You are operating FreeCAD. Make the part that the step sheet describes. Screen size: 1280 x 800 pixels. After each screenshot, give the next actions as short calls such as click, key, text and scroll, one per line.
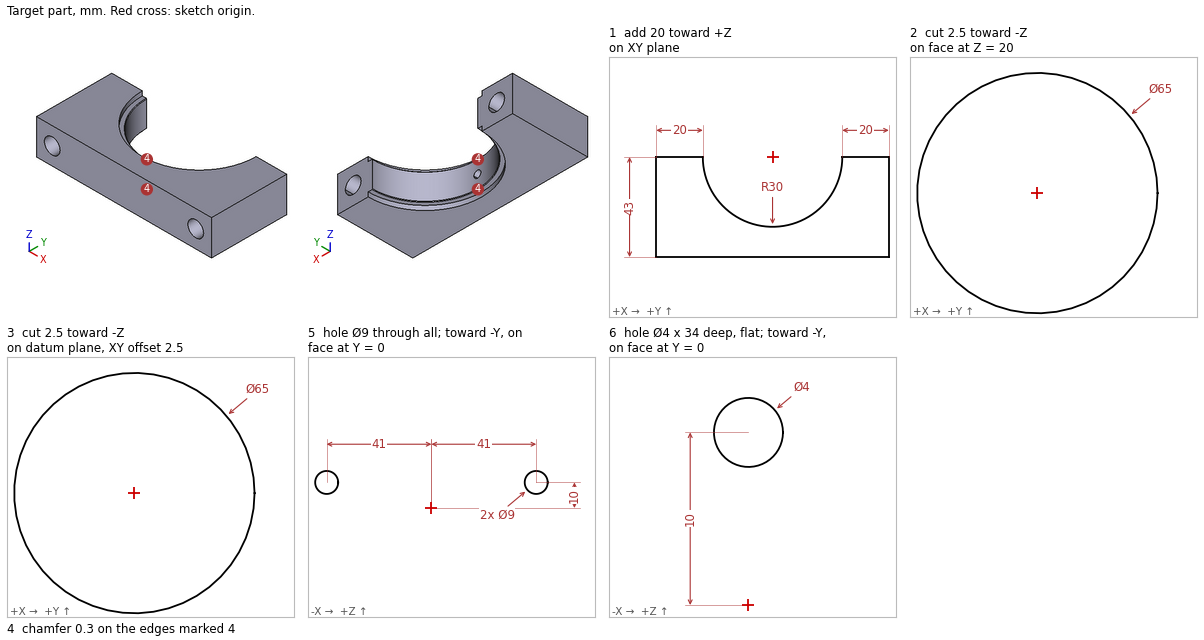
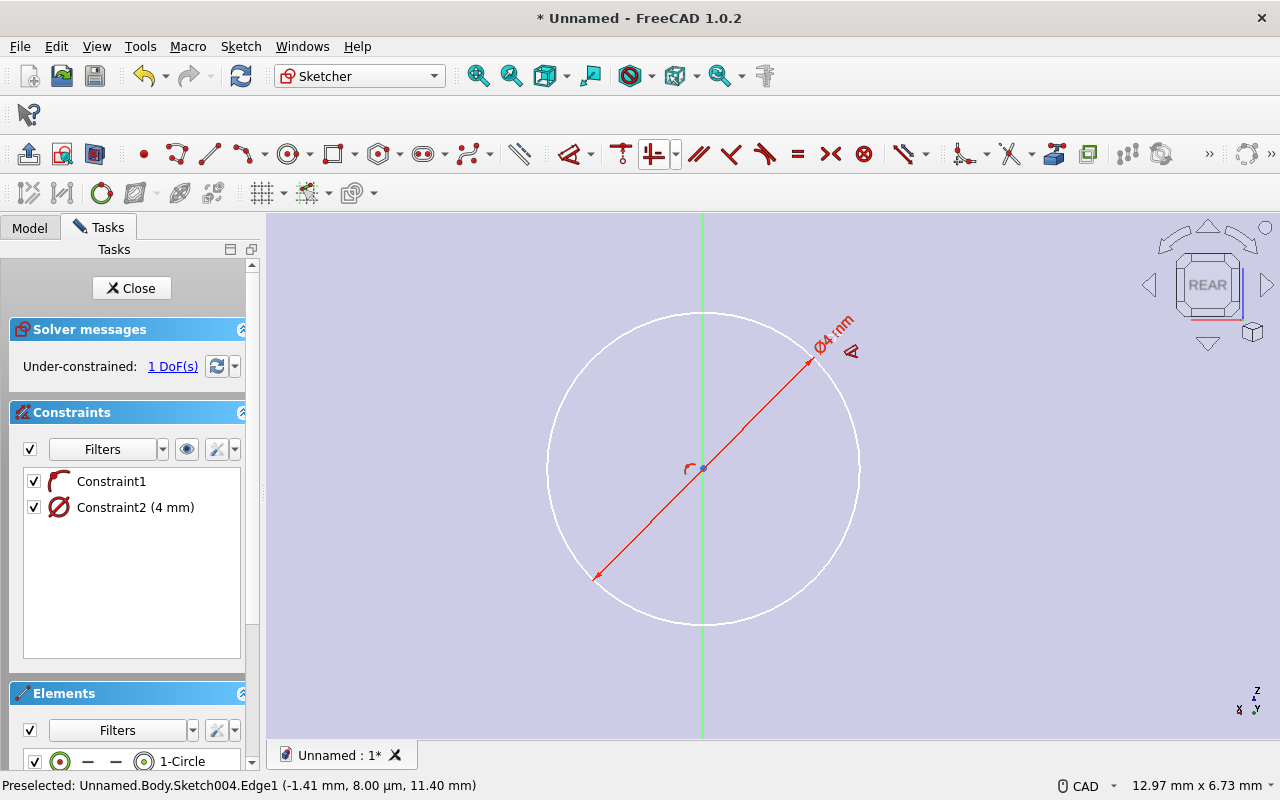
click(703, 469)
click(737, 590)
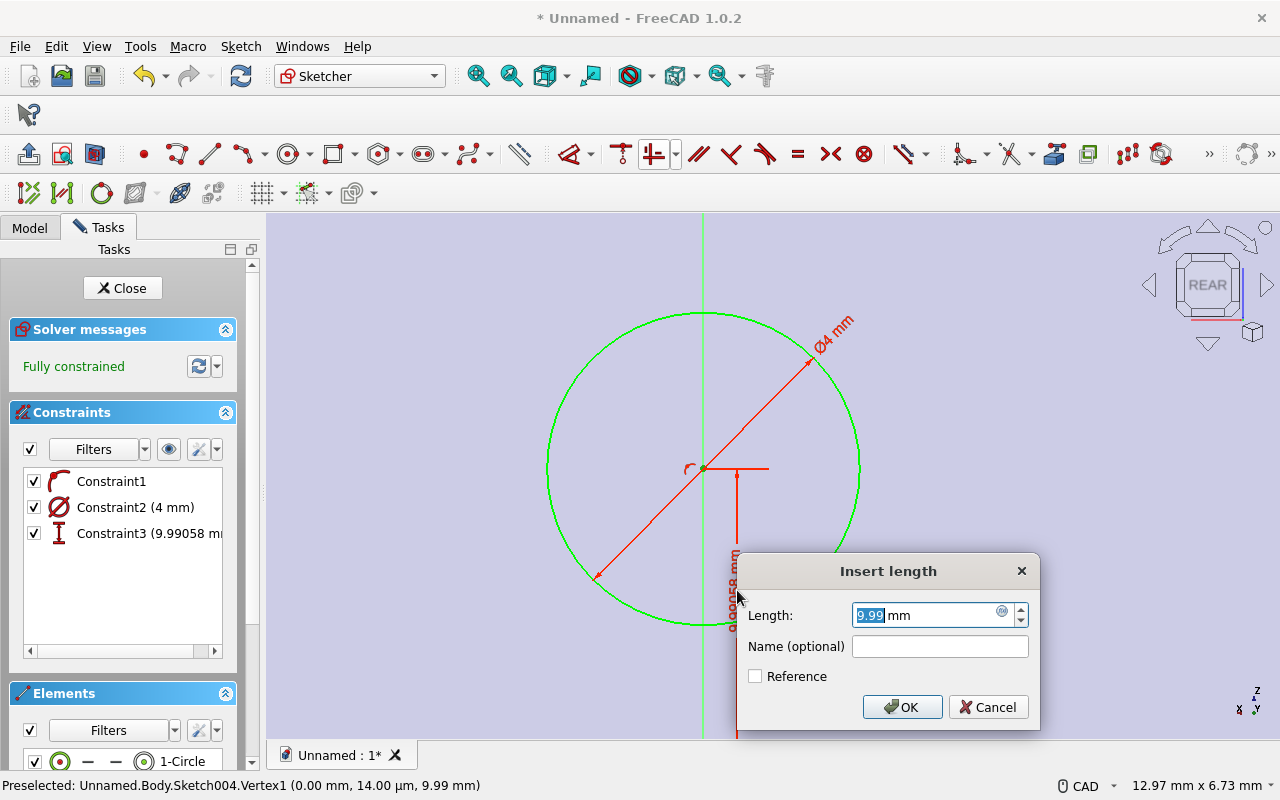
text(10)
key(Return)
key(Escape)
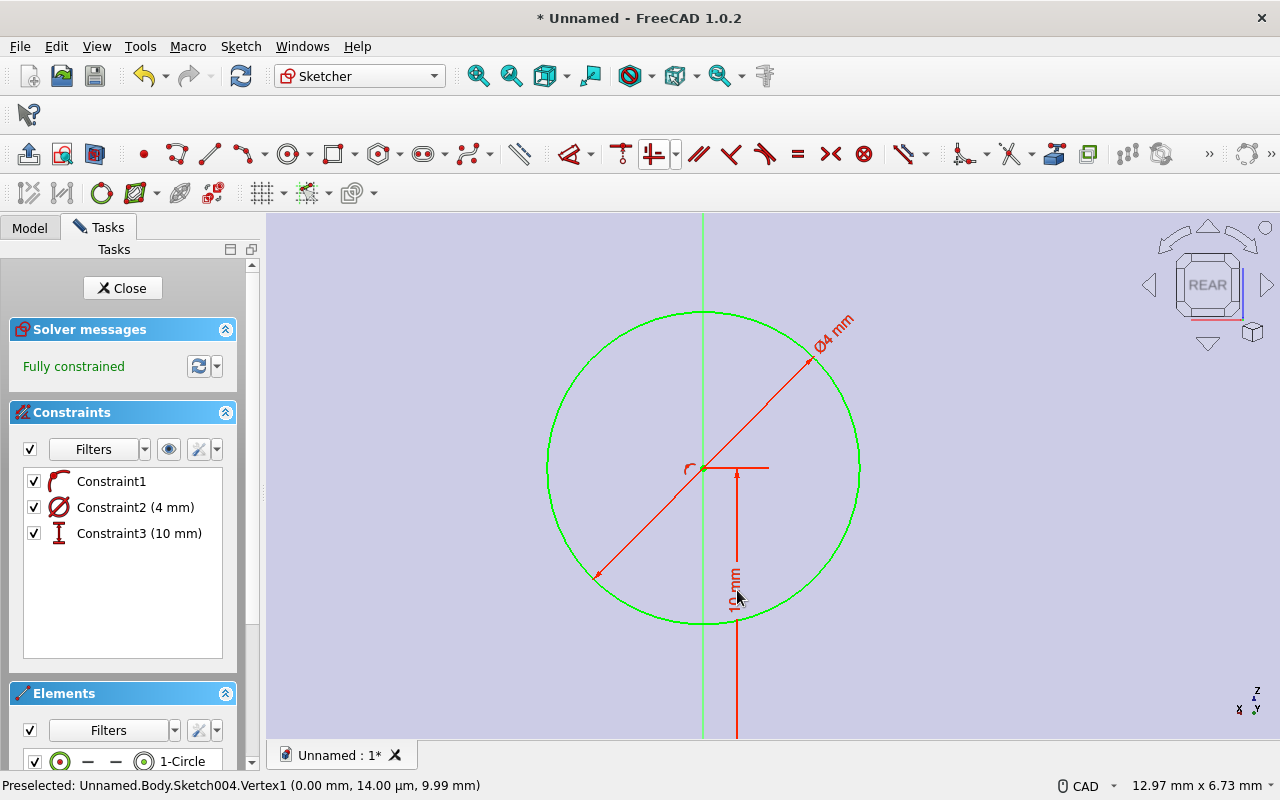
click(123, 288)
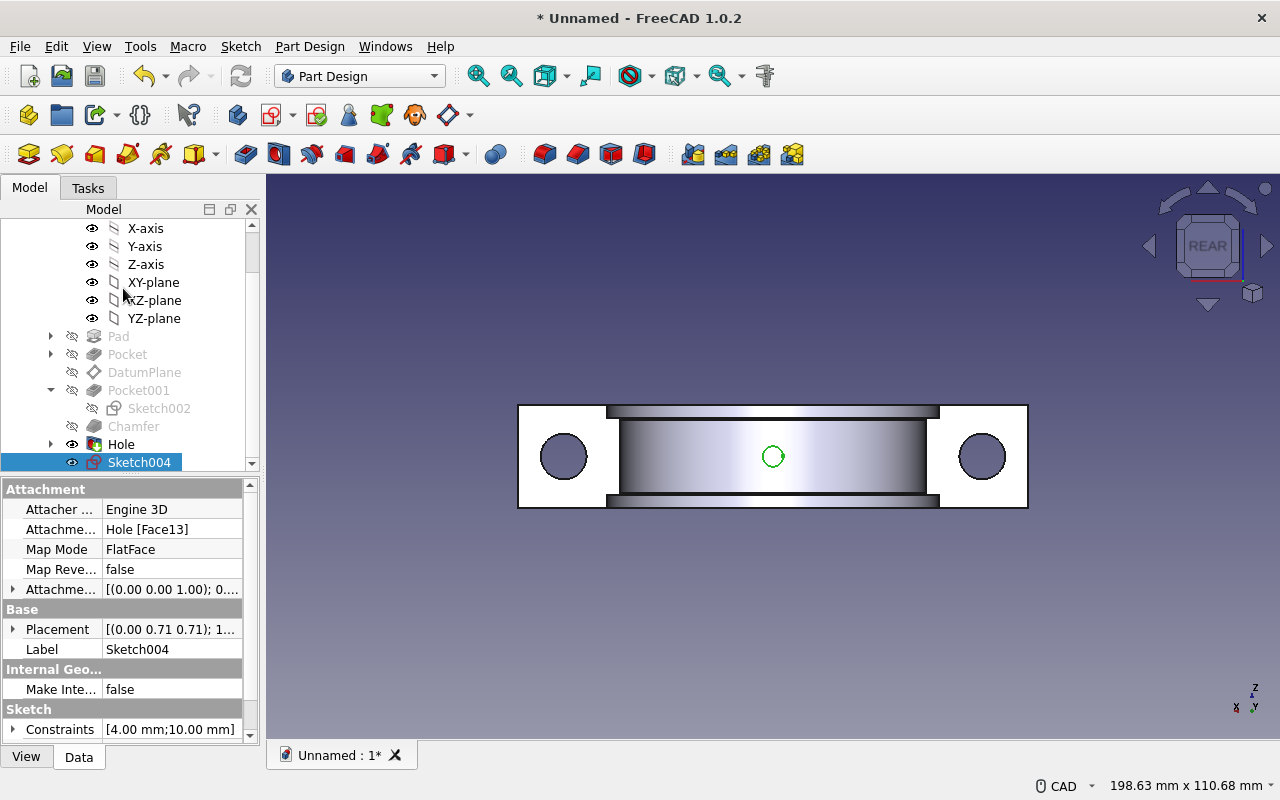
click(279, 154)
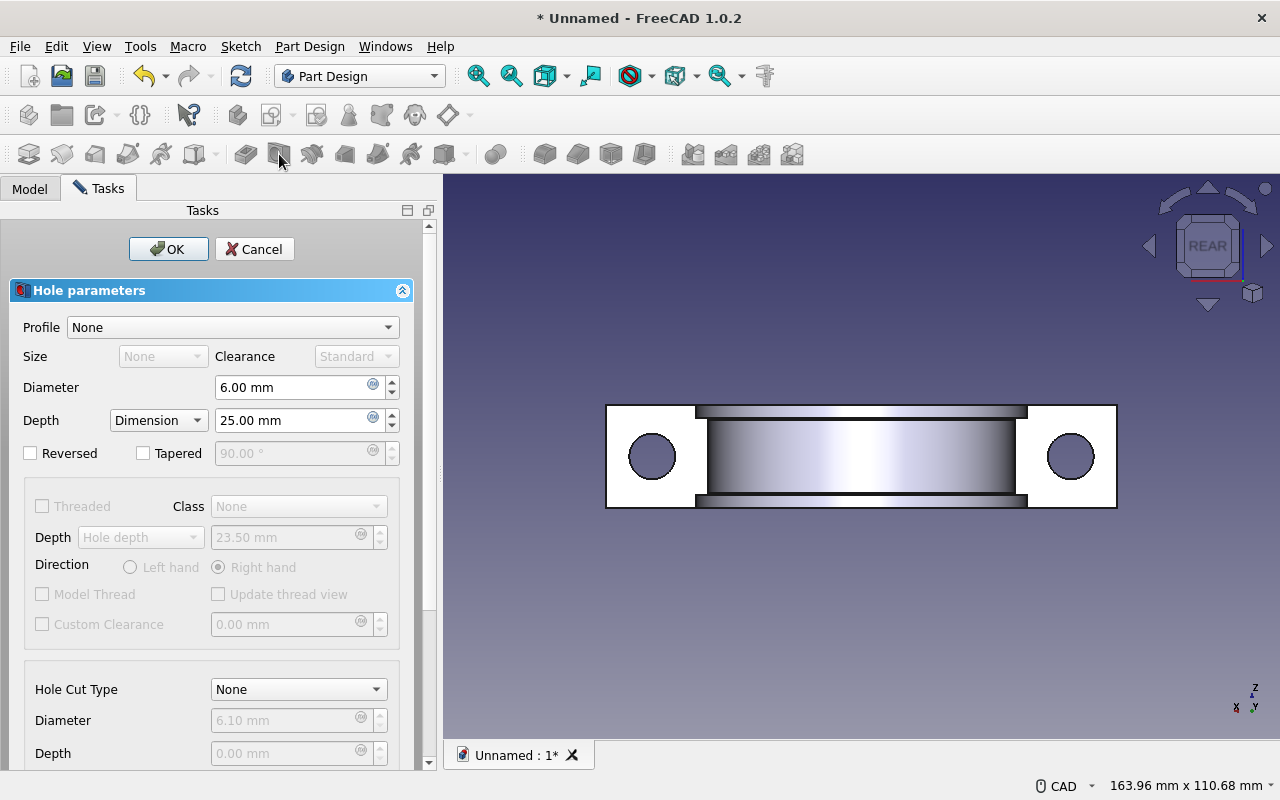
triple_click(300, 388)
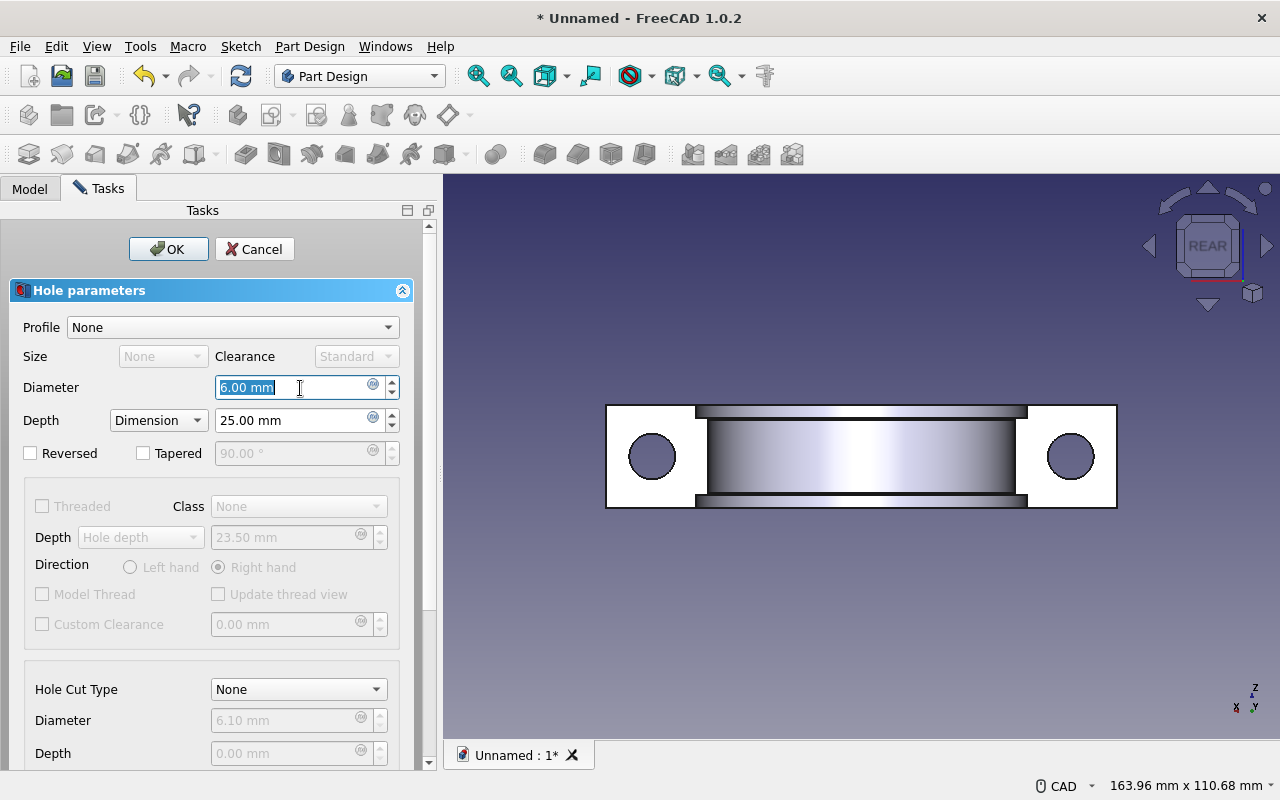
text(4)
key(Tab)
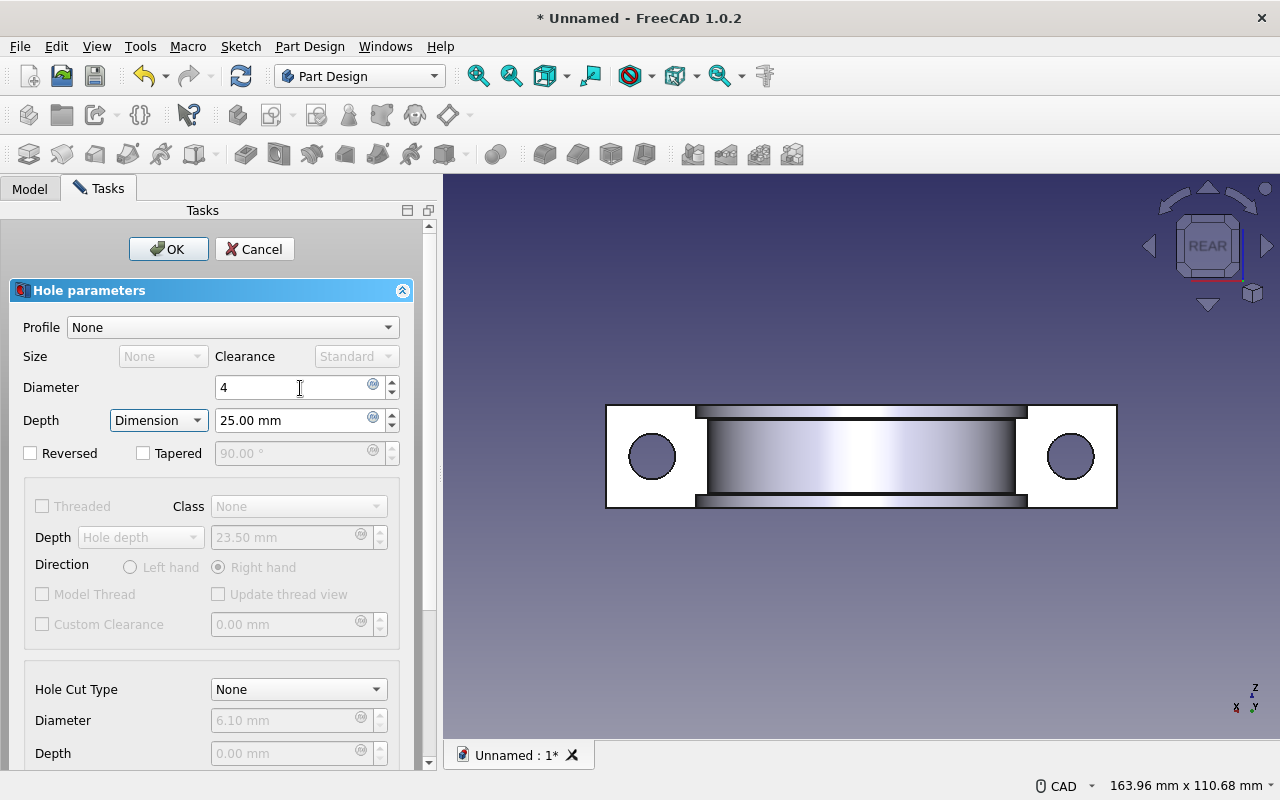
triple_click(300, 420)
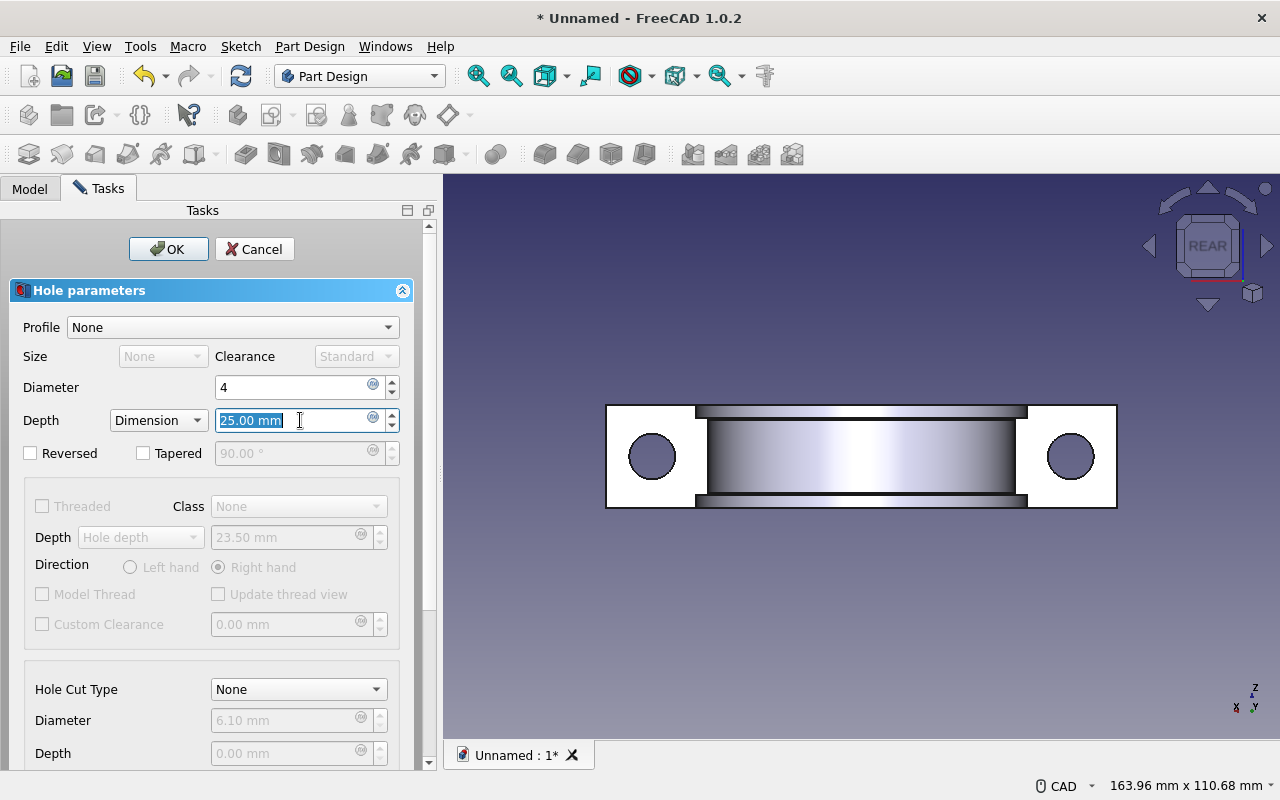
text(34)
key(Tab)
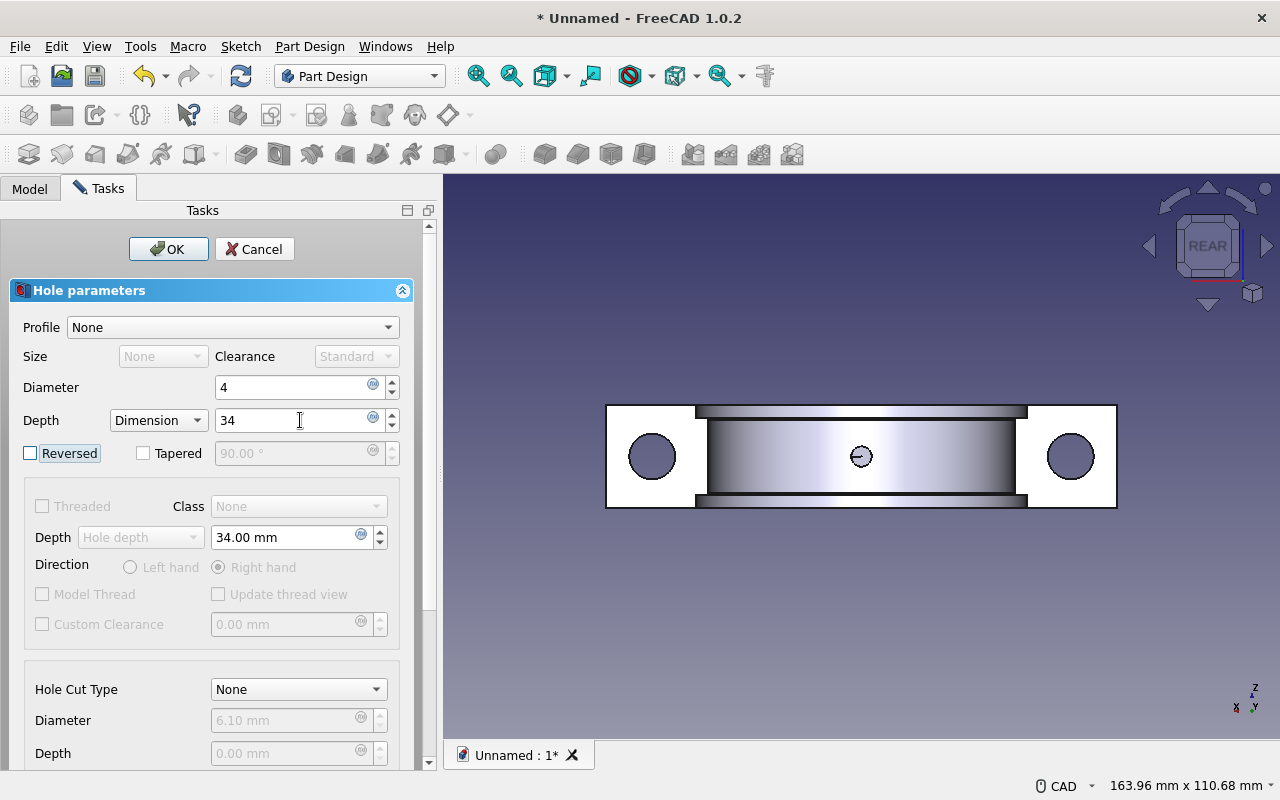
scroll(429, 495, down, 3)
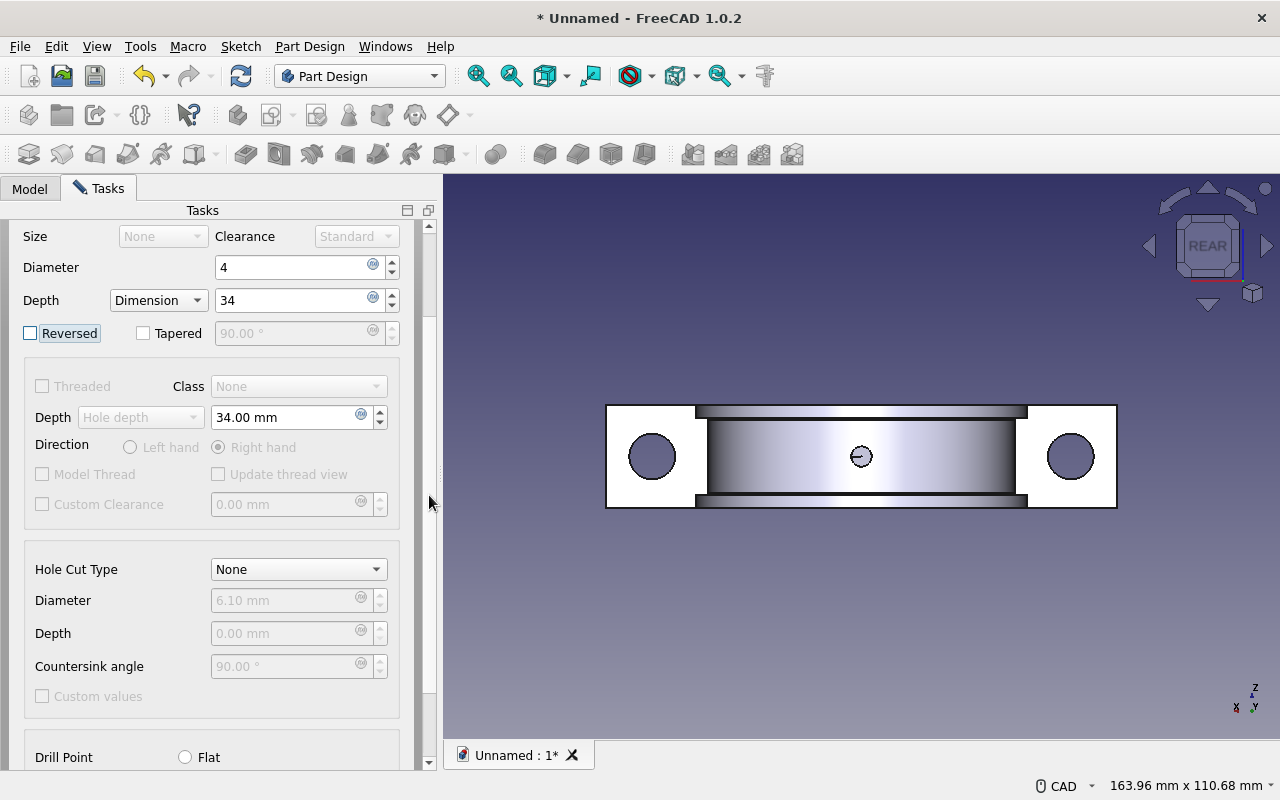
click(186, 695)